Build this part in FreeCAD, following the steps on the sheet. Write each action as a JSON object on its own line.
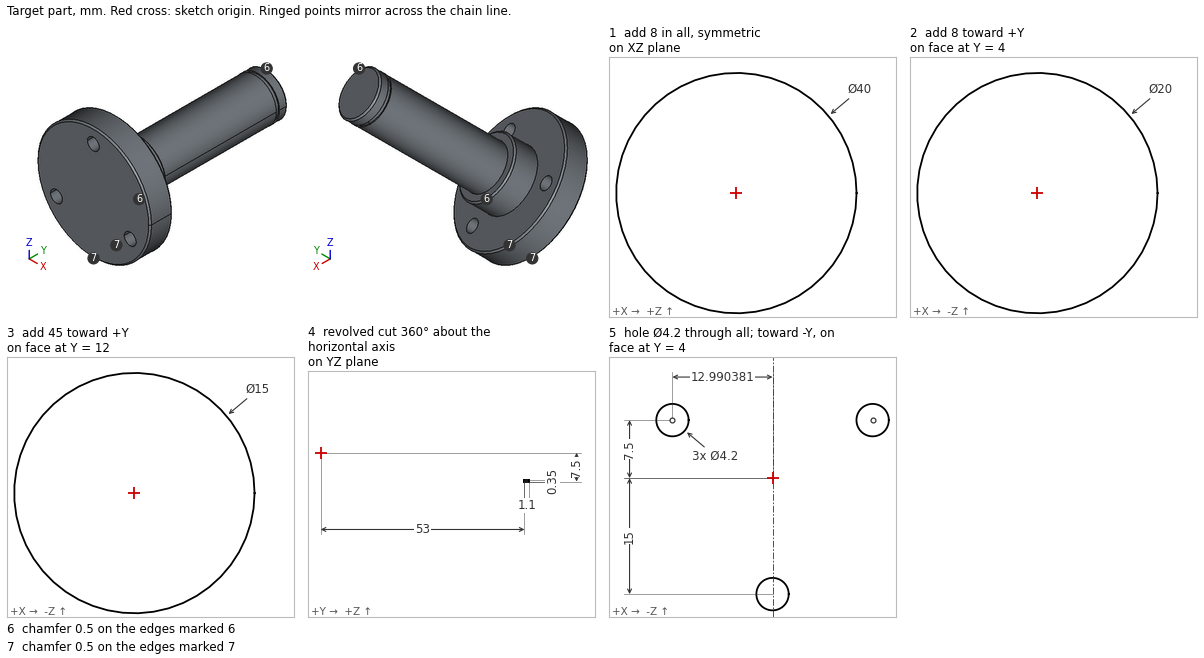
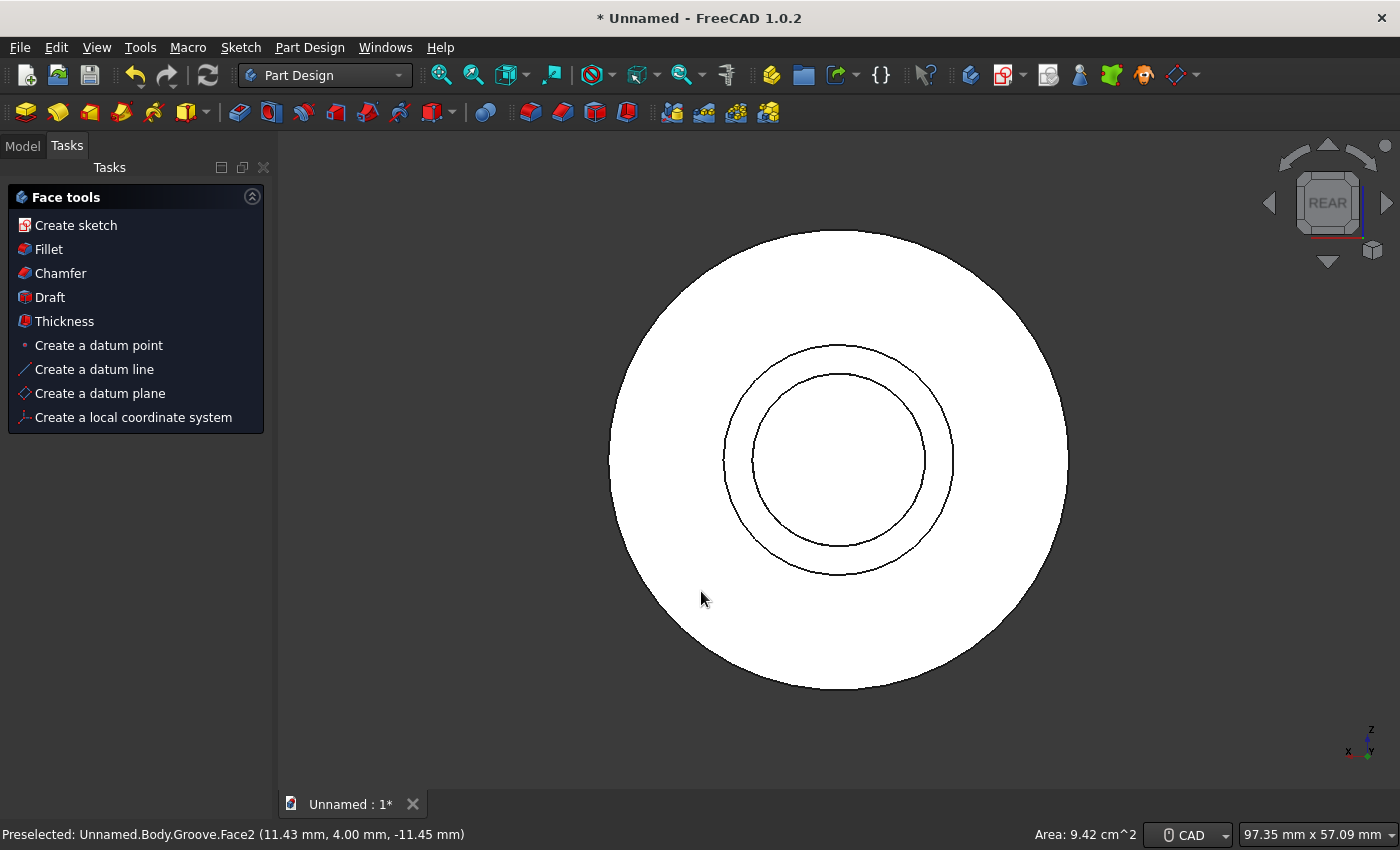
{"action": "left_click", "coordinate": [1004, 76]}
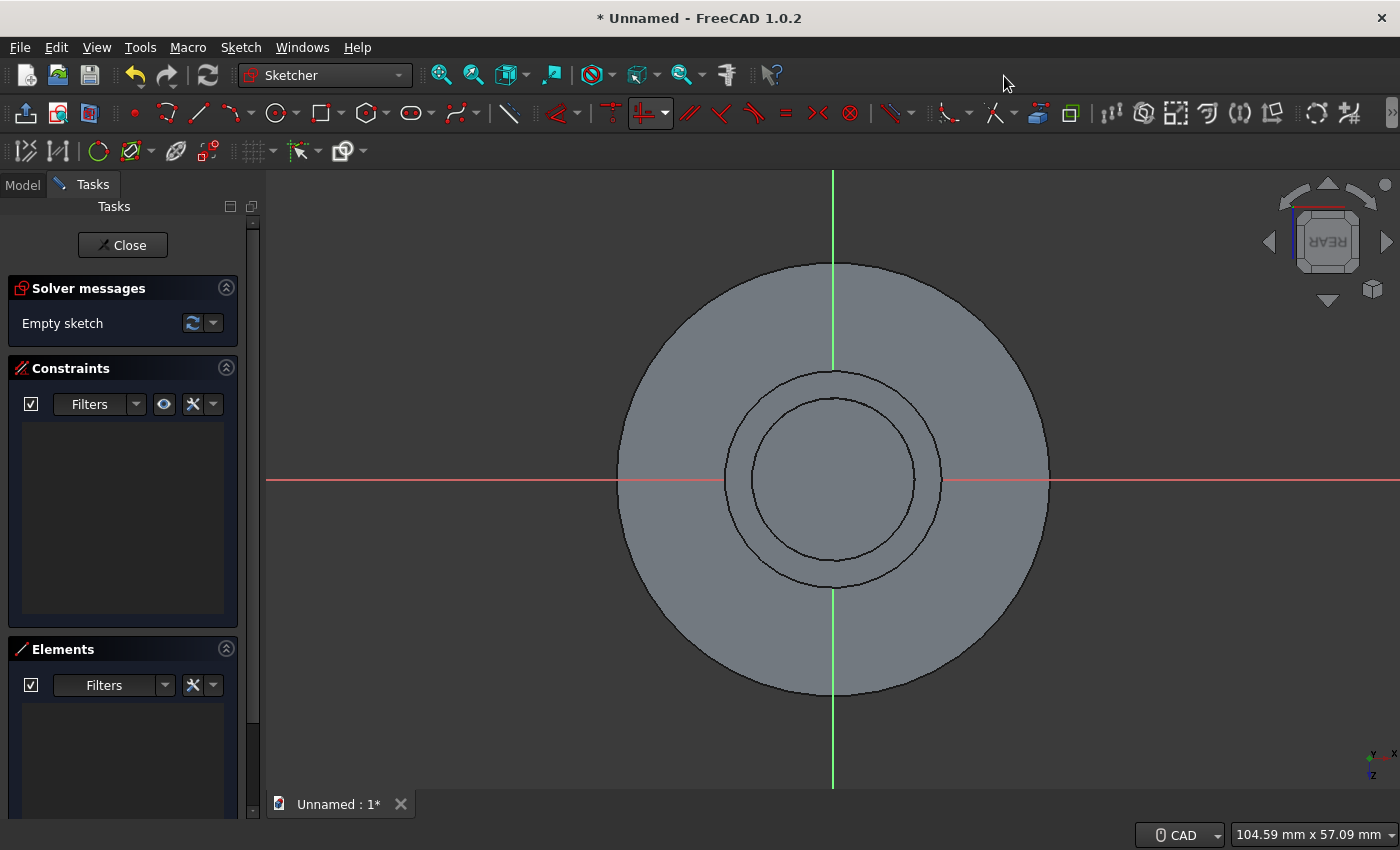
{"action": "left_click", "coordinate": [90, 114]}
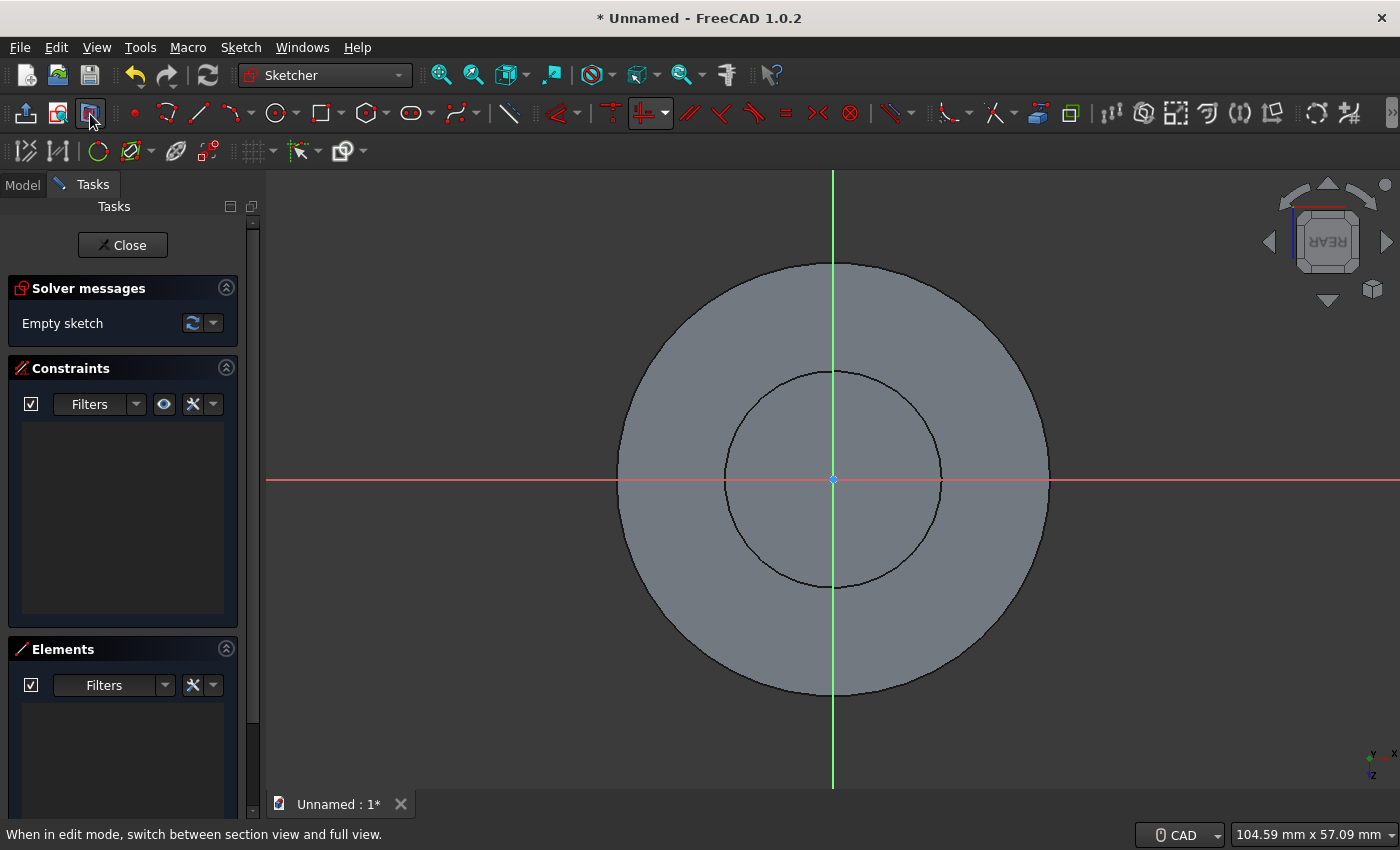
{"action": "scroll", "coordinate": [973, 603], "scroll_direction": "up", "scroll_amount": 2}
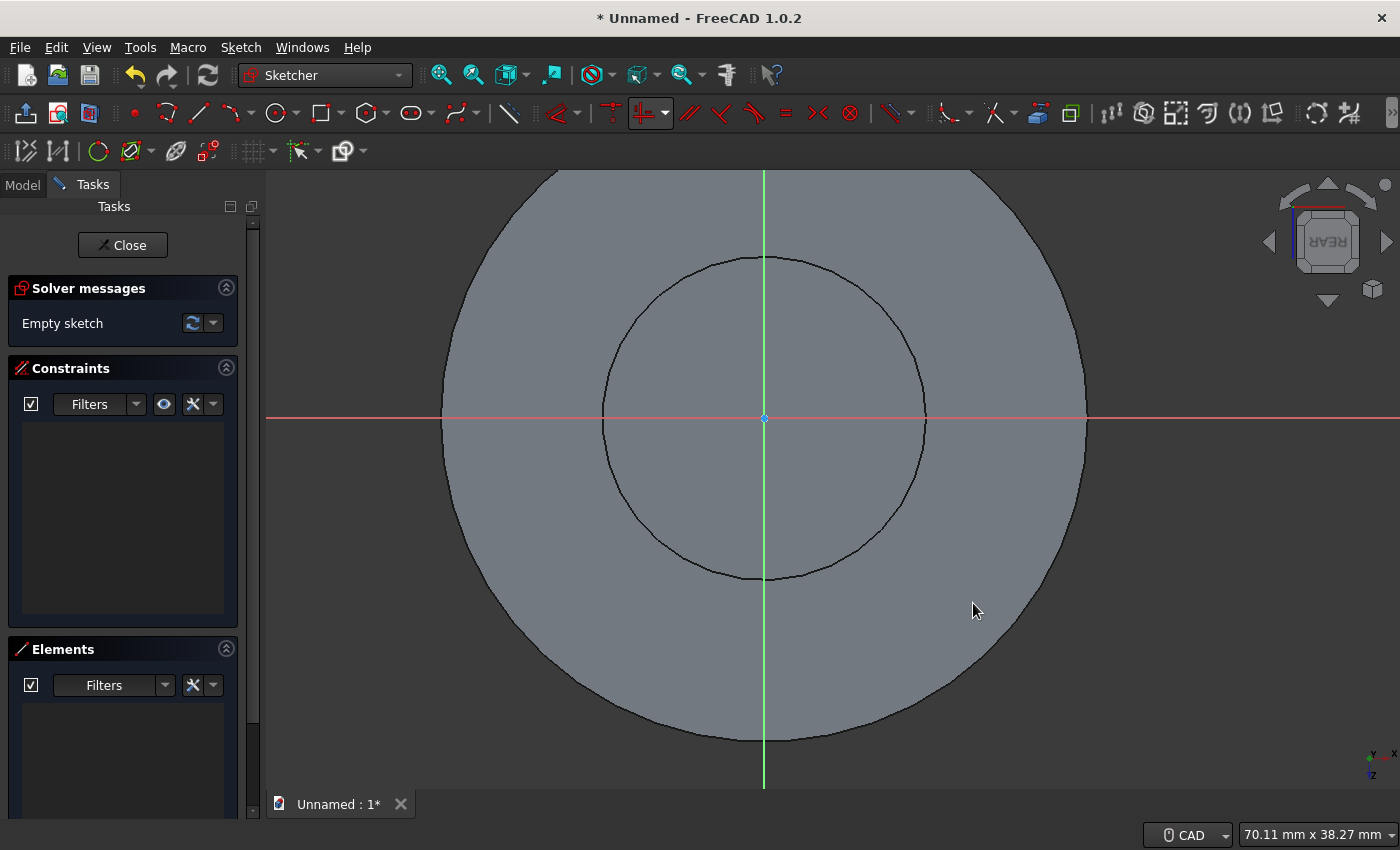
{"action": "left_click", "coordinate": [276, 114]}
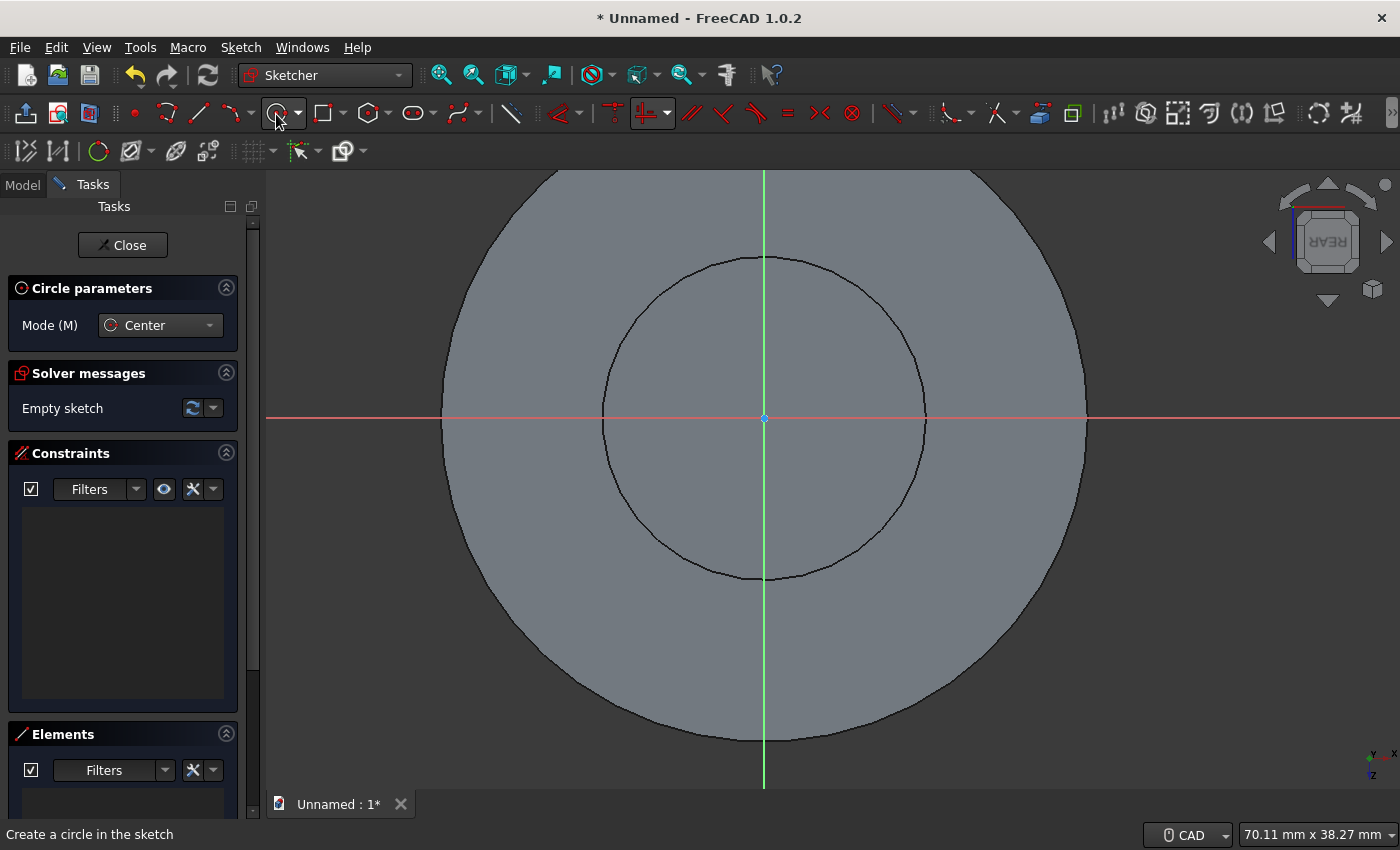
{"action": "left_click", "coordinate": [554, 297]}
{"action": "mouse_move", "coordinate": [578, 273]}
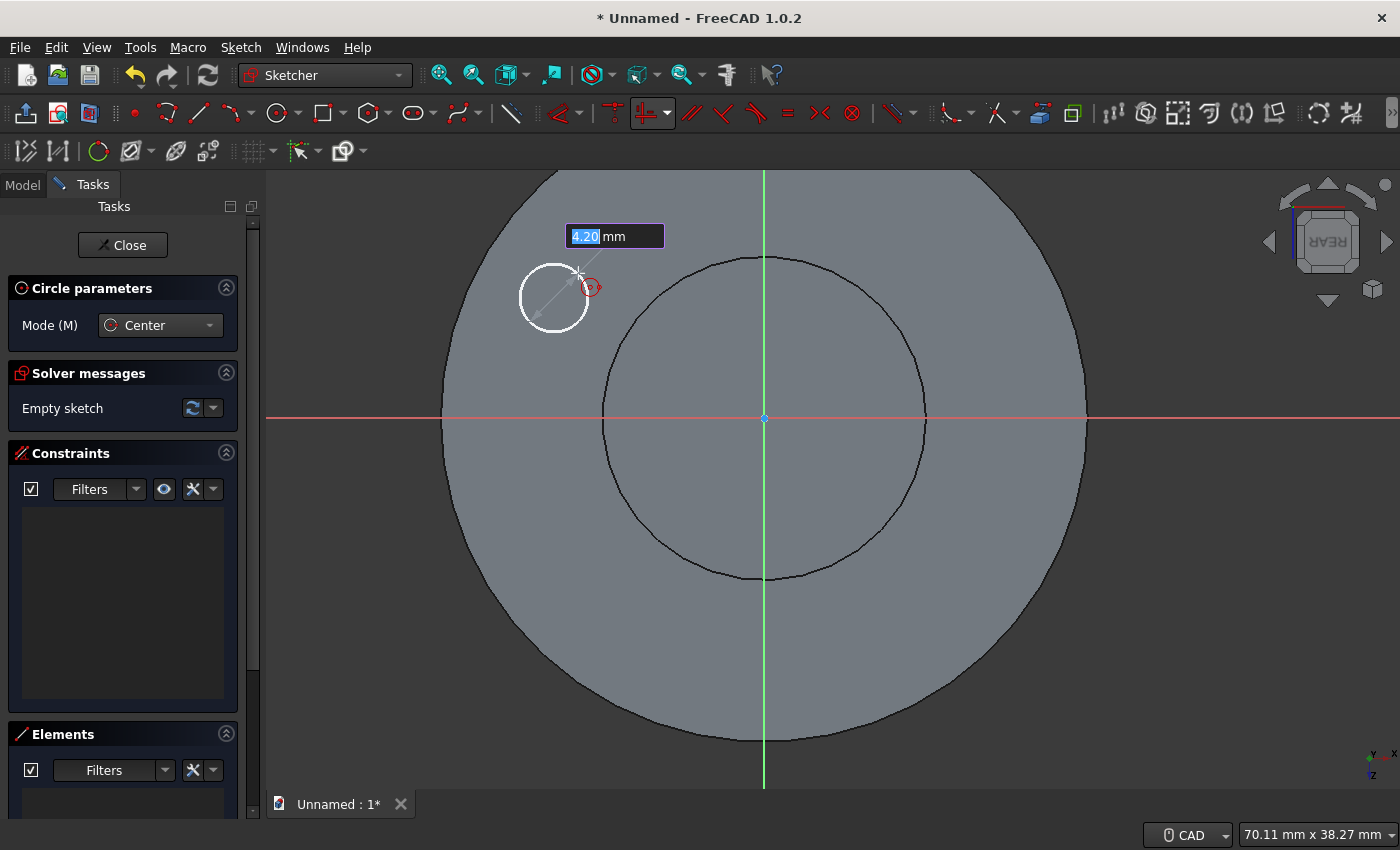
{"action": "type", "text": "4.2"}
{"action": "key", "text": "Return"}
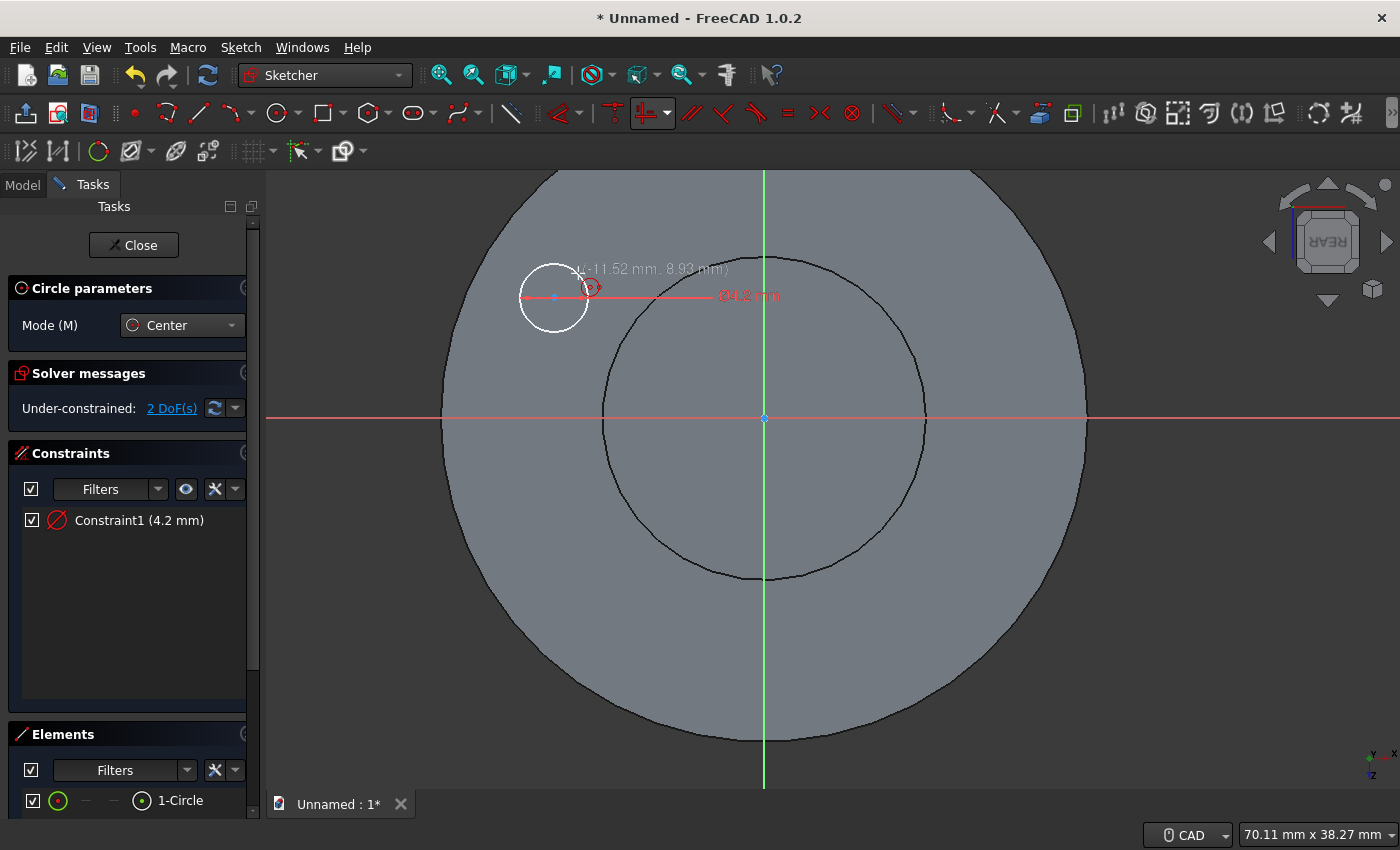
{"action": "left_click", "coordinate": [974, 297]}
{"action": "mouse_move", "coordinate": [998, 273]}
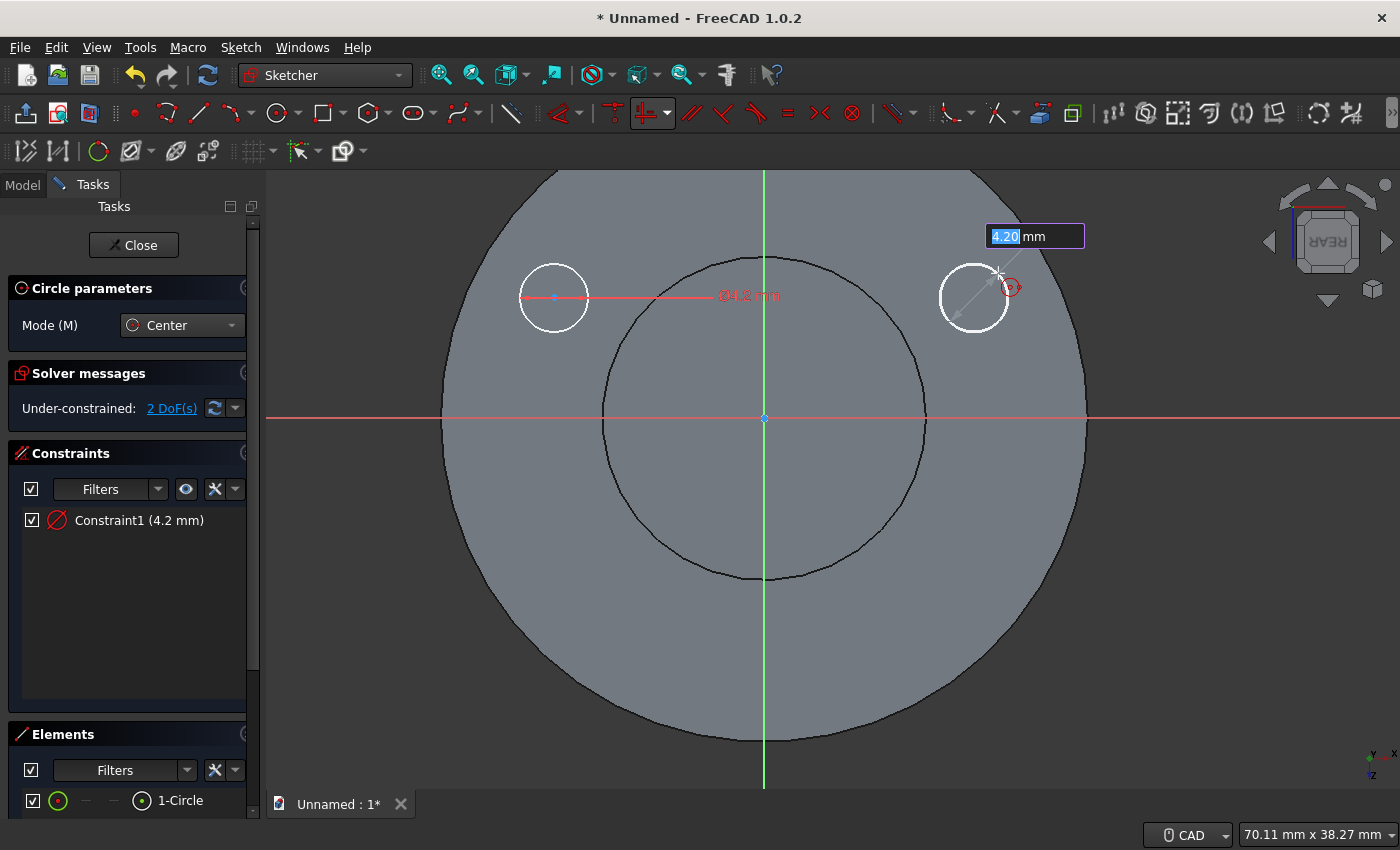
{"action": "type", "text": "4.2"}
{"action": "key", "text": "Return"}